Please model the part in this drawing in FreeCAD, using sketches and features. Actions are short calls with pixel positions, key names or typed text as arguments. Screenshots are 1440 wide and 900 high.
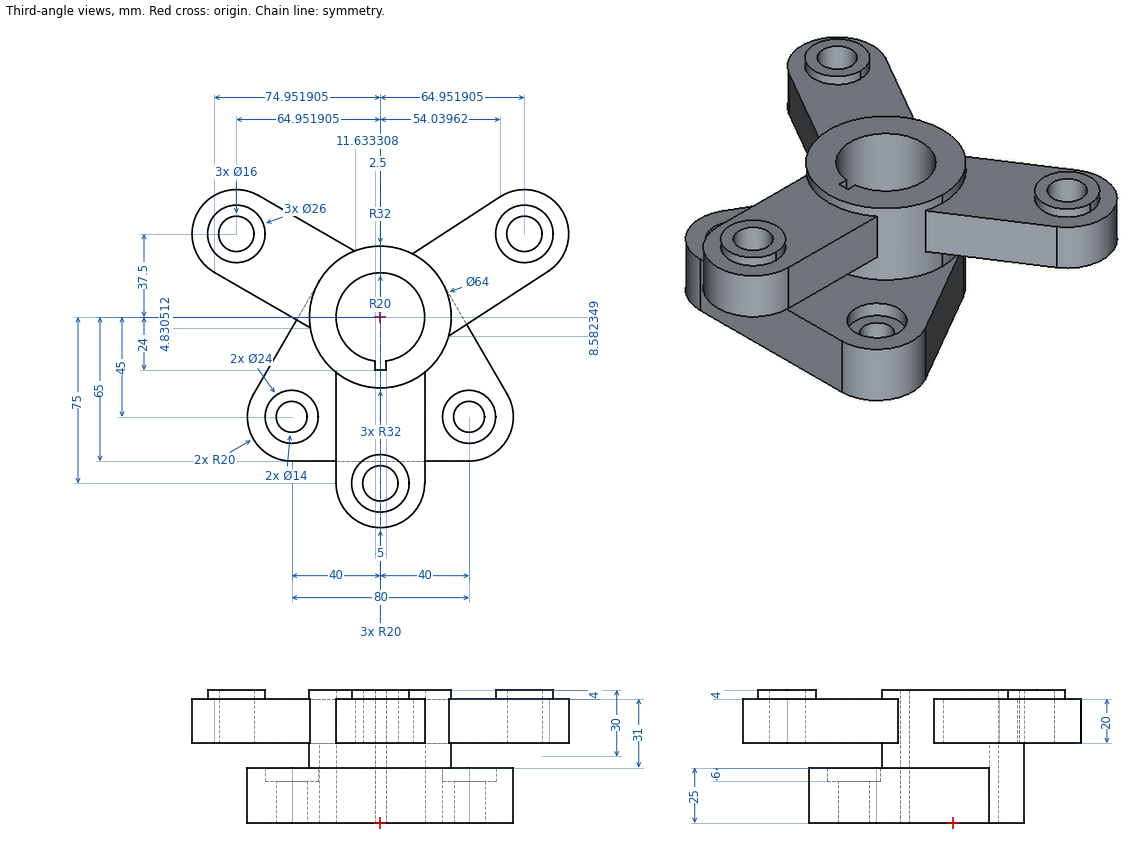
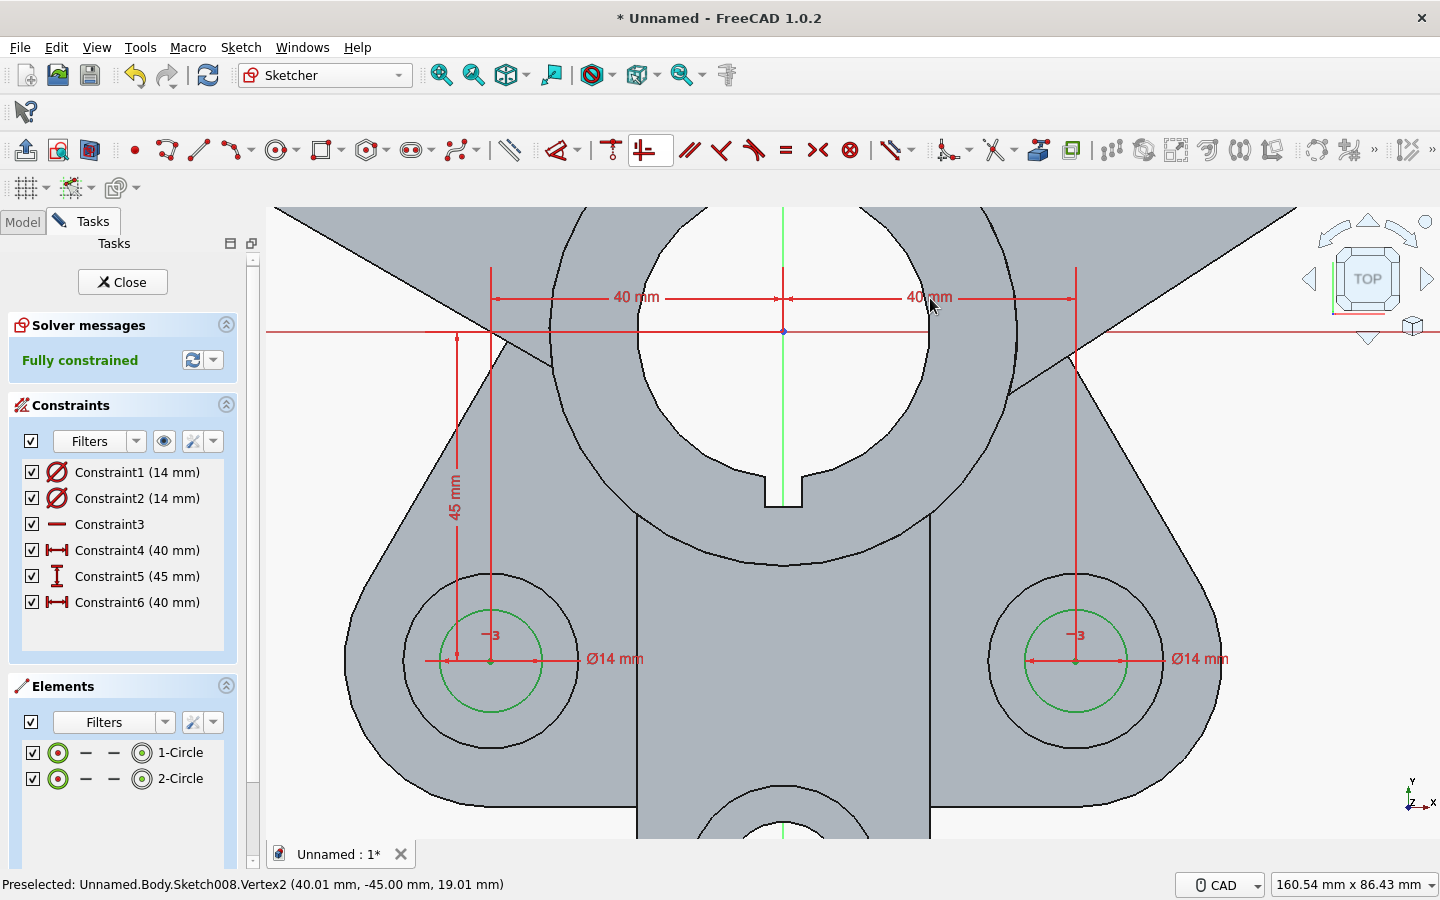
click(123, 282)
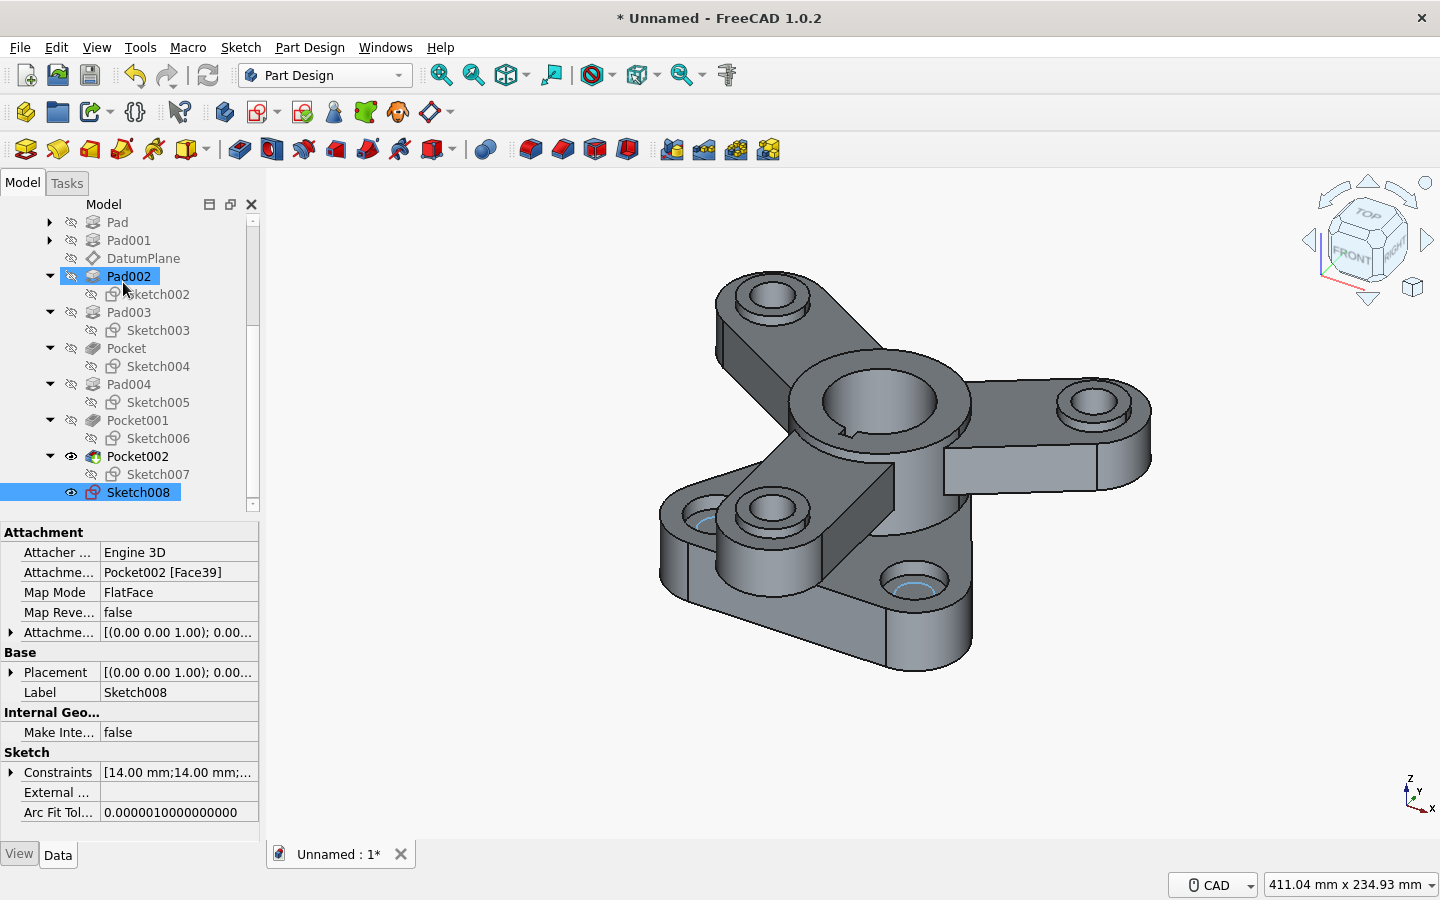
click(240, 150)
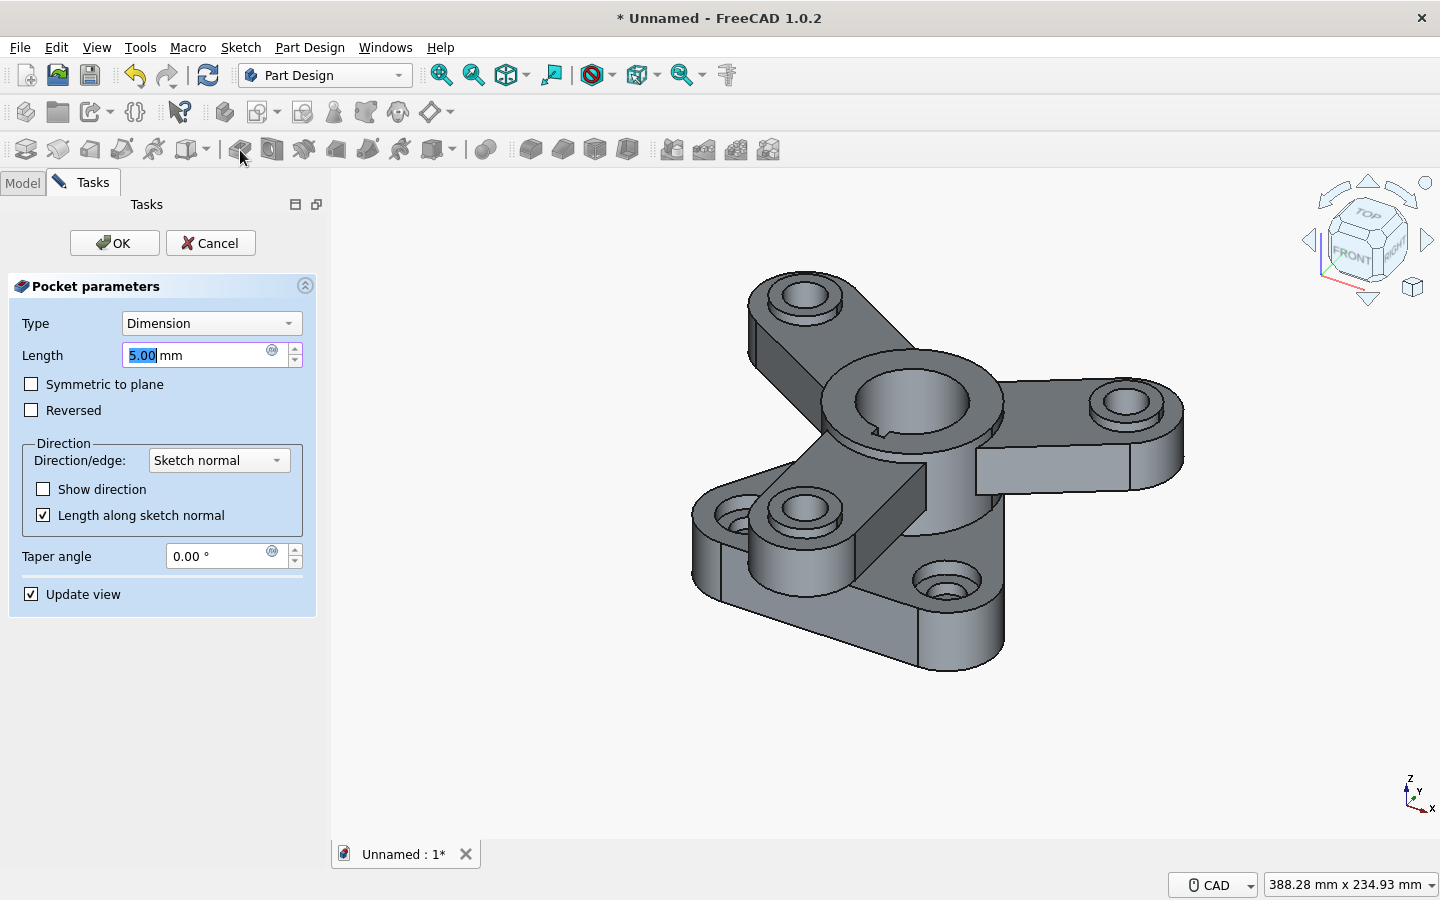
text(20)
key(Tab)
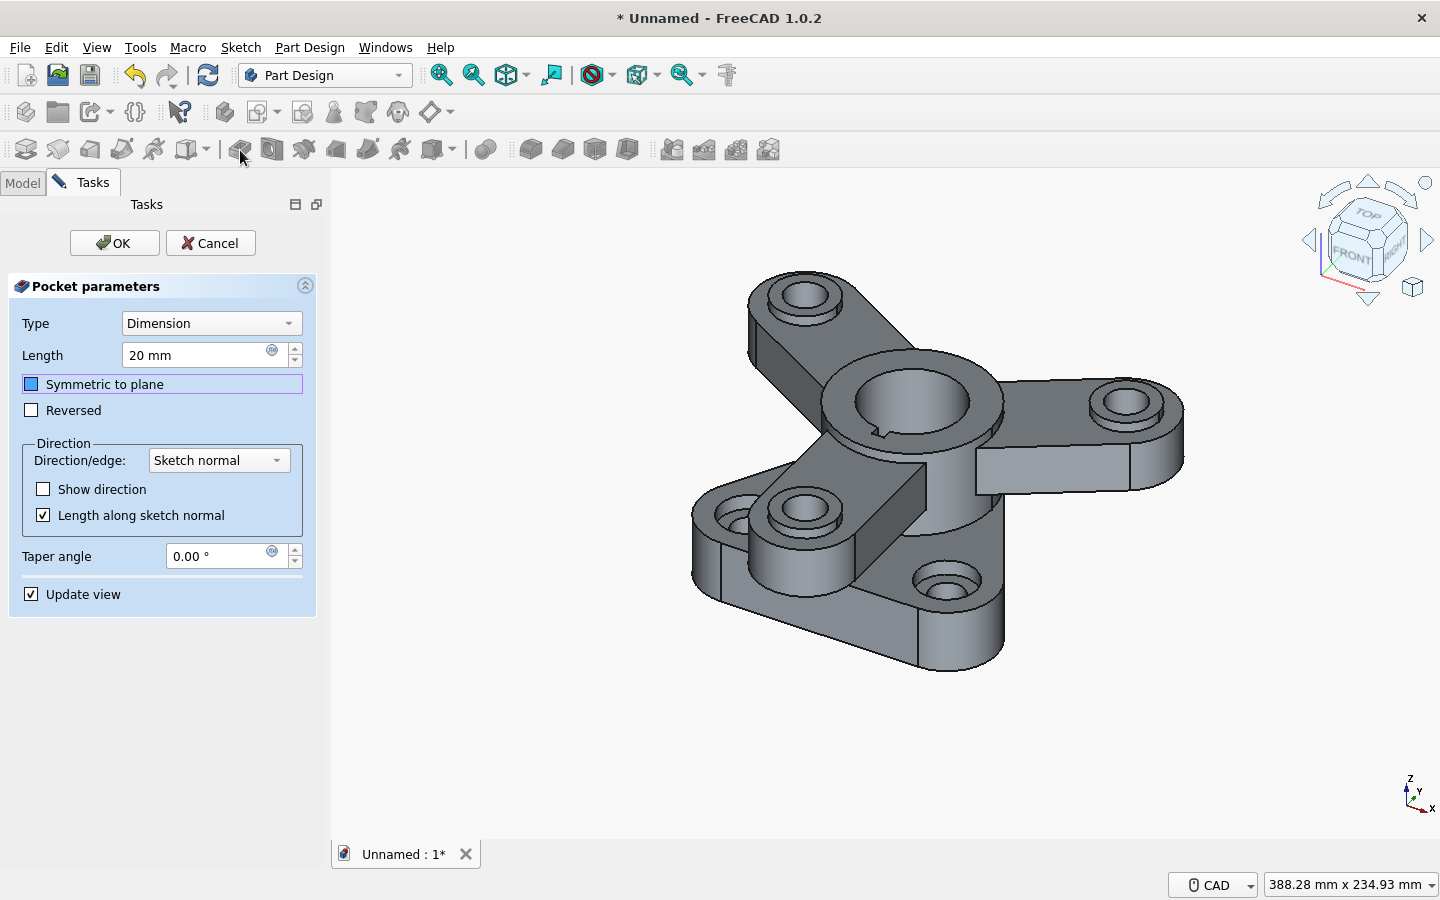
click(115, 243)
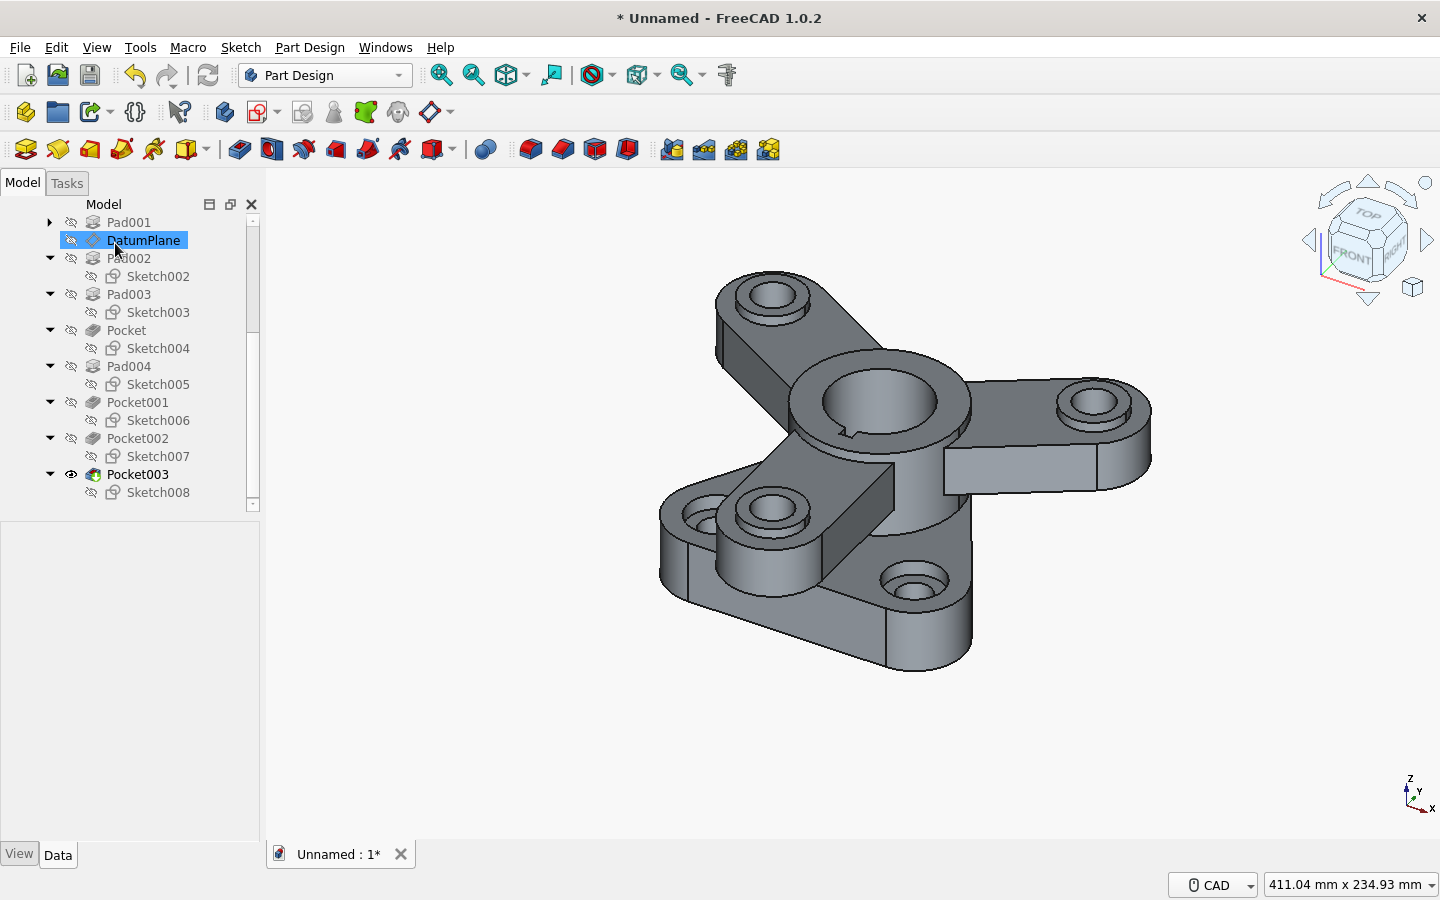
key(0)